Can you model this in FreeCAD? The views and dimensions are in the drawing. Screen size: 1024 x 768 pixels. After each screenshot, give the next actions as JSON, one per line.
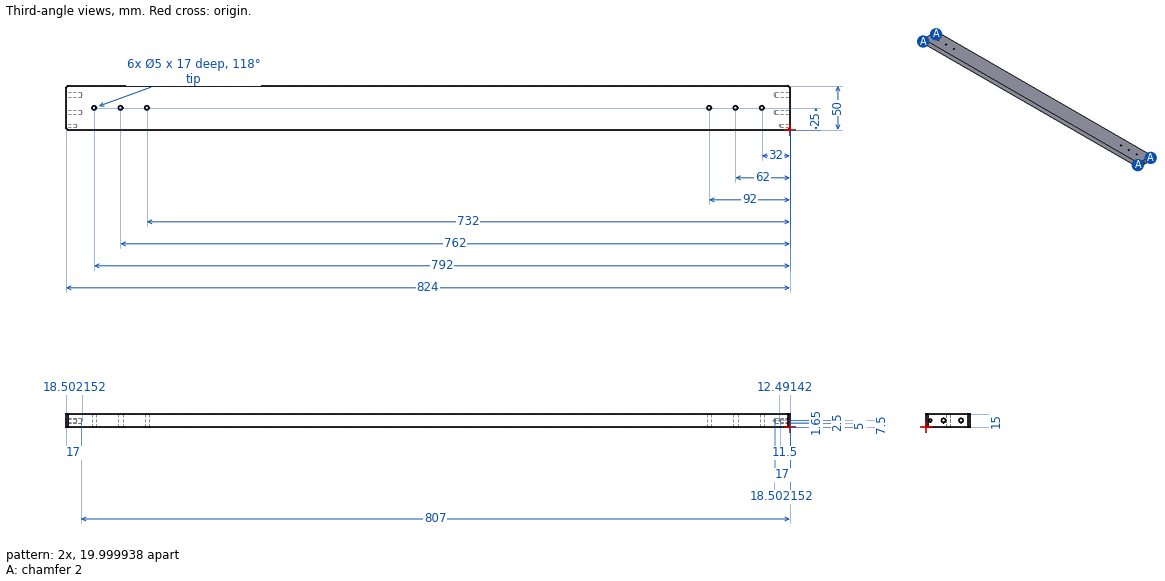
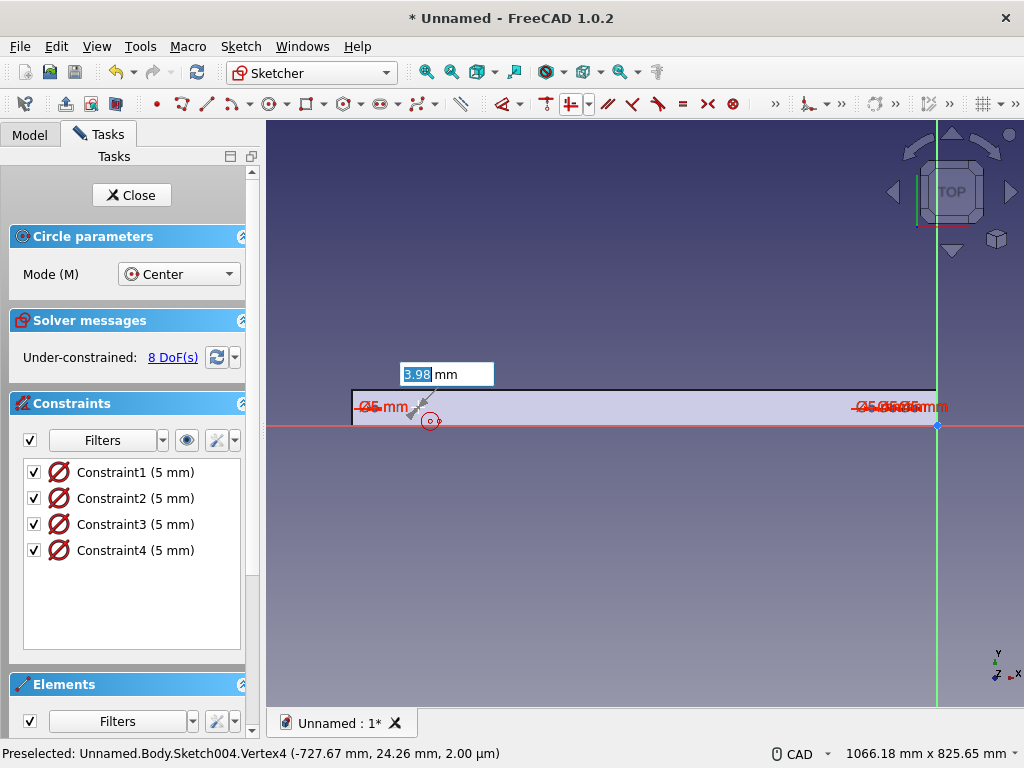
{"action": "type", "text": "5"}
{"action": "key", "text": "Return"}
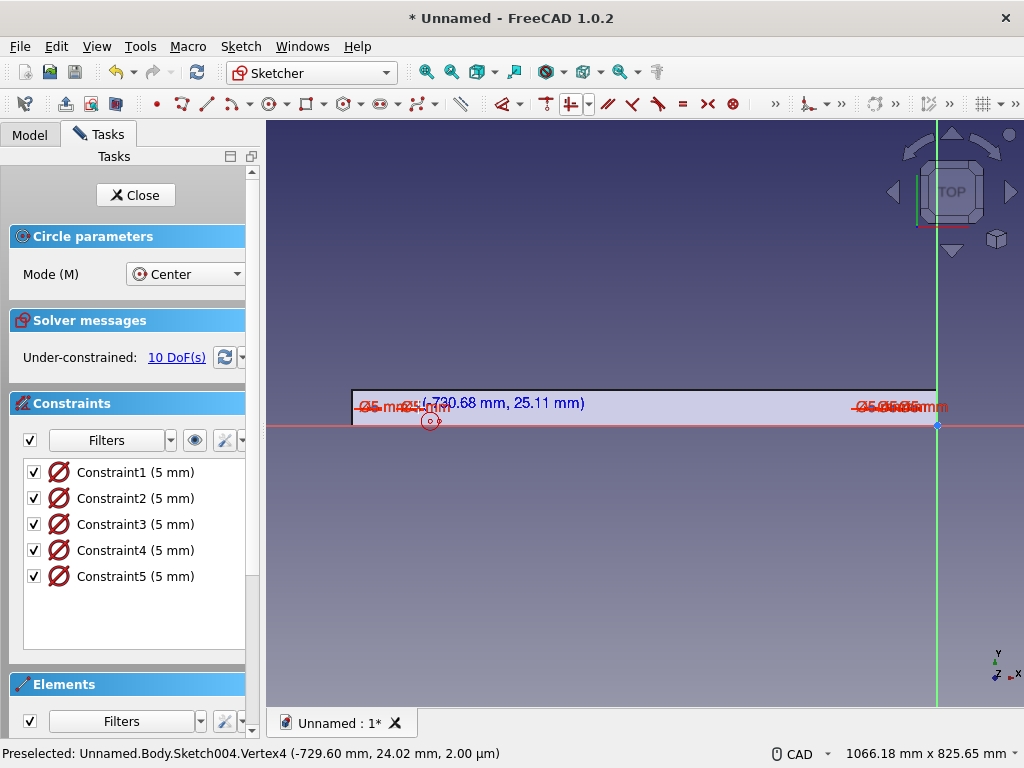
{"action": "scroll", "coordinate": [396, 408], "scroll_direction": "up", "scroll_amount": 13}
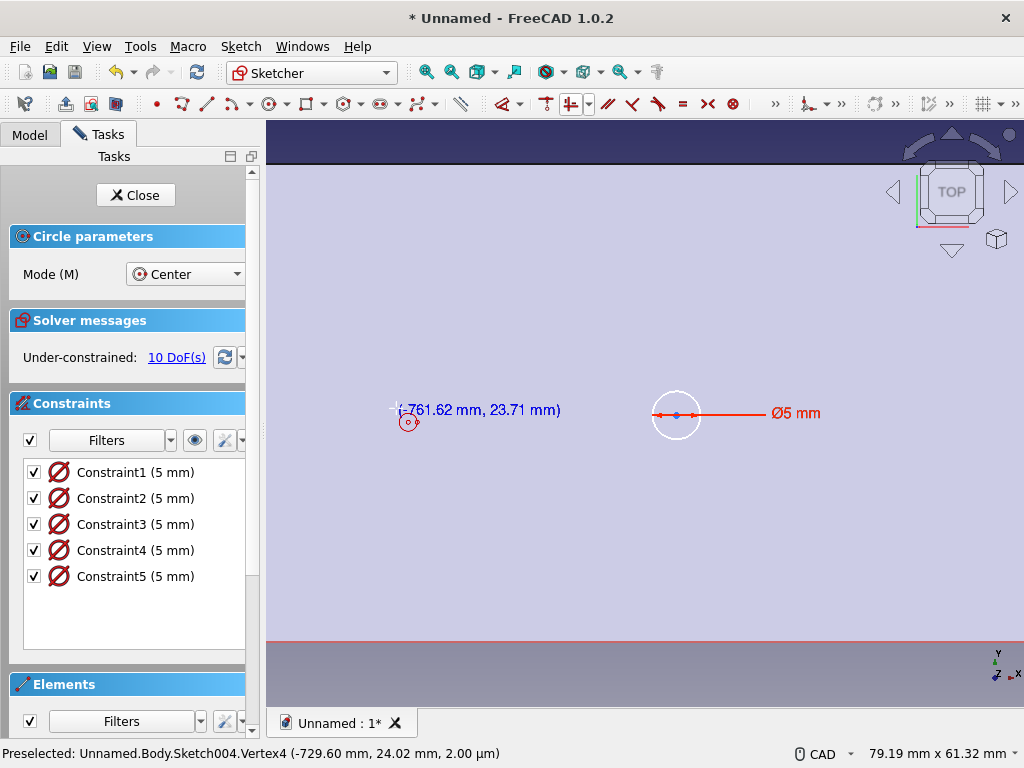
{"action": "scroll", "coordinate": [403, 408], "scroll_direction": "down", "scroll_amount": 15}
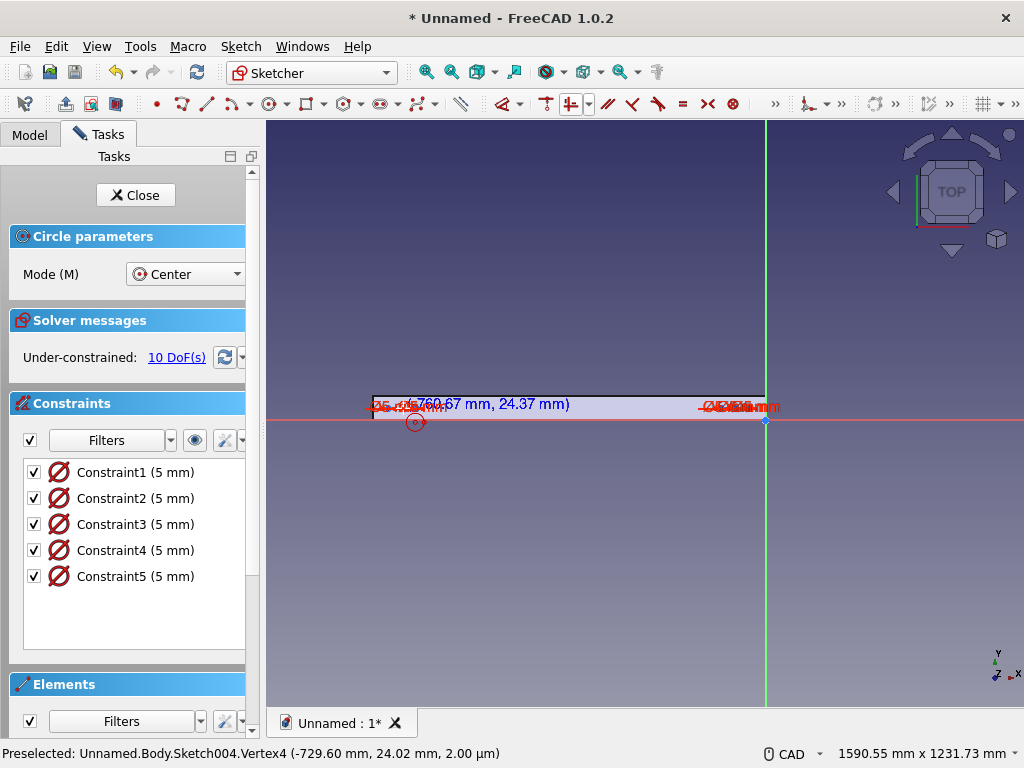
{"action": "scroll", "coordinate": [403, 408], "scroll_direction": "up", "scroll_amount": 2}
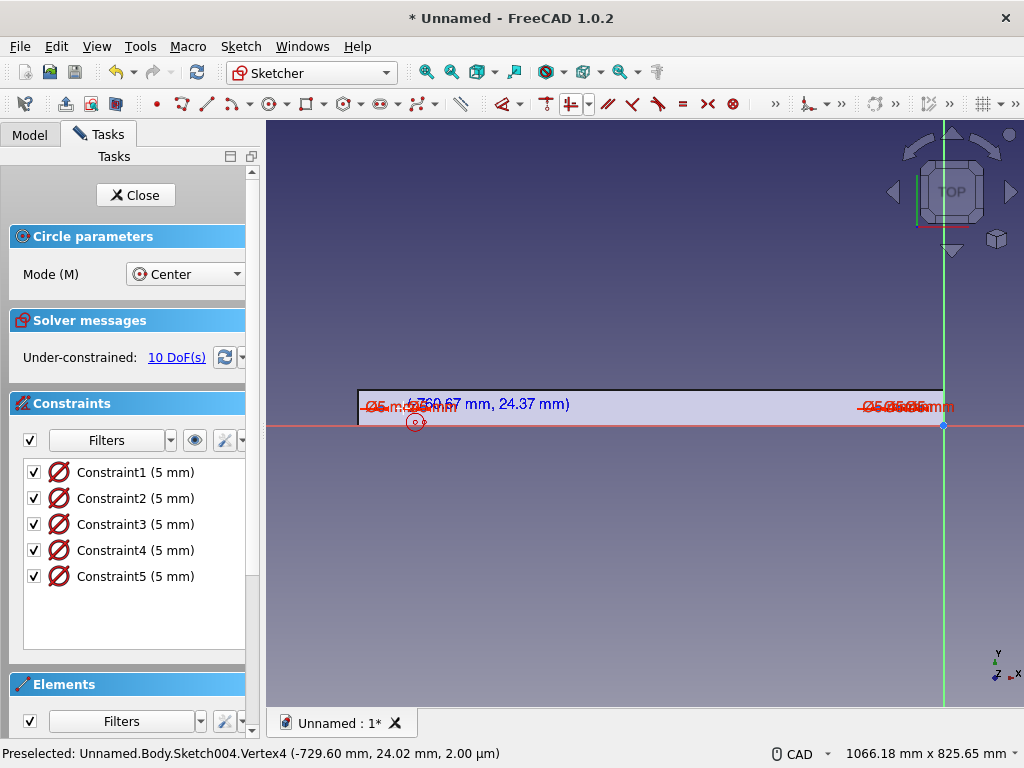
{"action": "left_click", "coordinate": [402, 408]}
{"action": "mouse_move", "coordinate": [403, 407]}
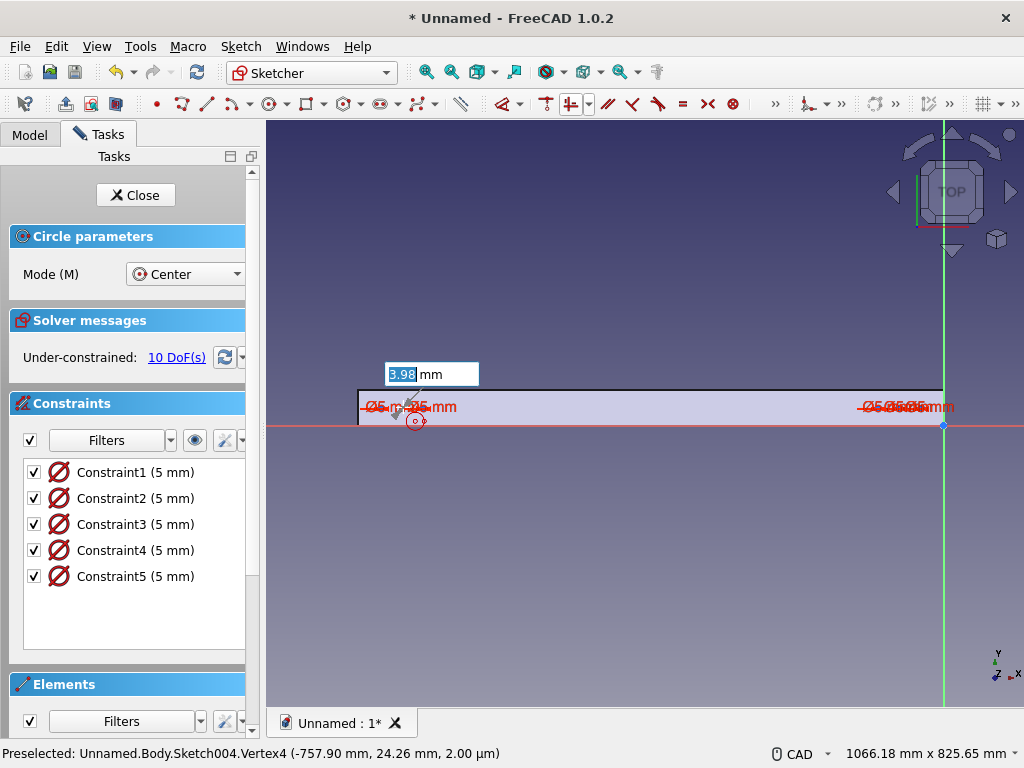
{"action": "type", "text": "5"}
{"action": "key", "text": "Return"}
{"action": "key", "text": "Escape"}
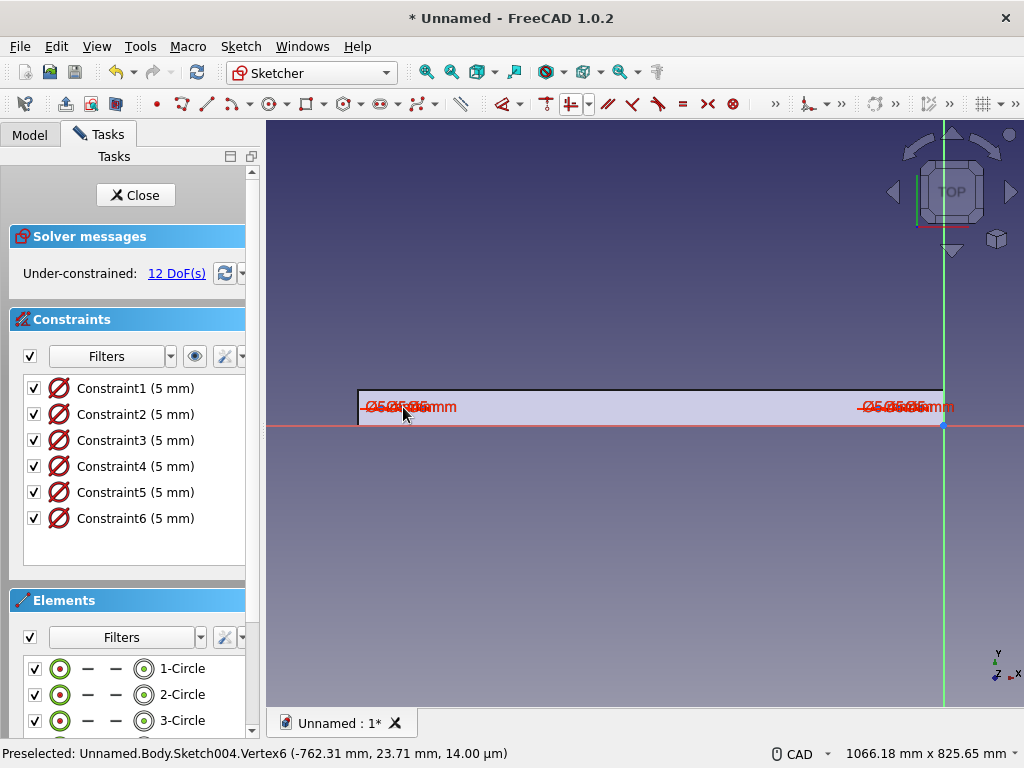
{"action": "left_click", "coordinate": [381, 409]}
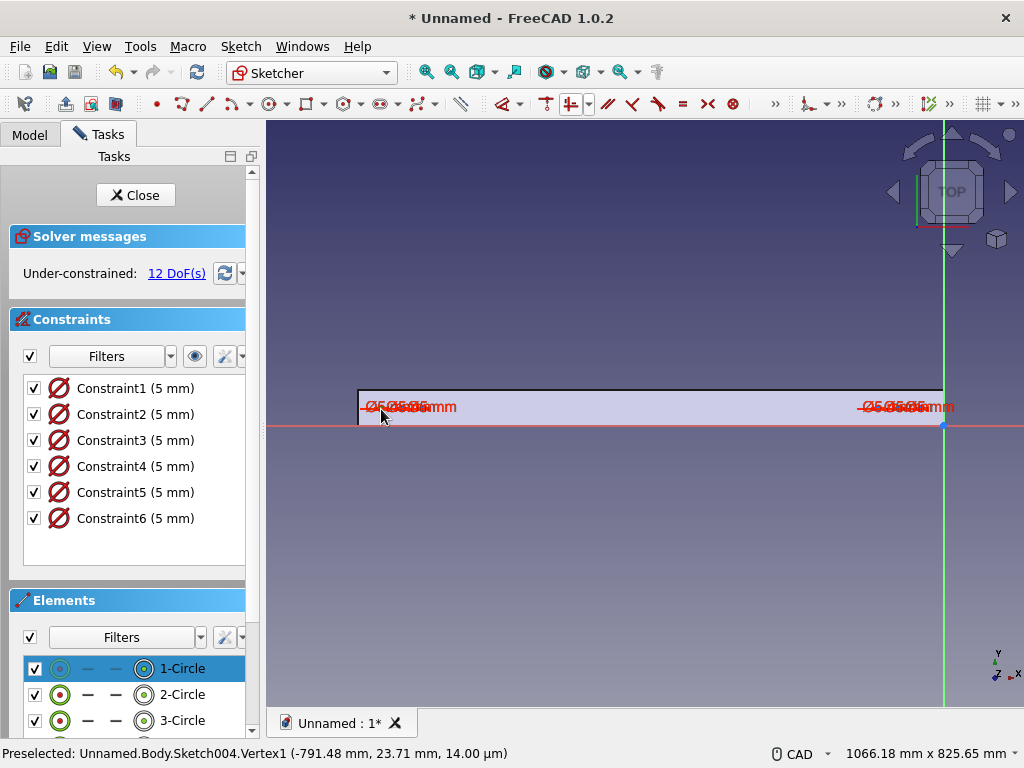
{"action": "scroll", "coordinate": [404, 408], "scroll_direction": "down", "scroll_amount": 2}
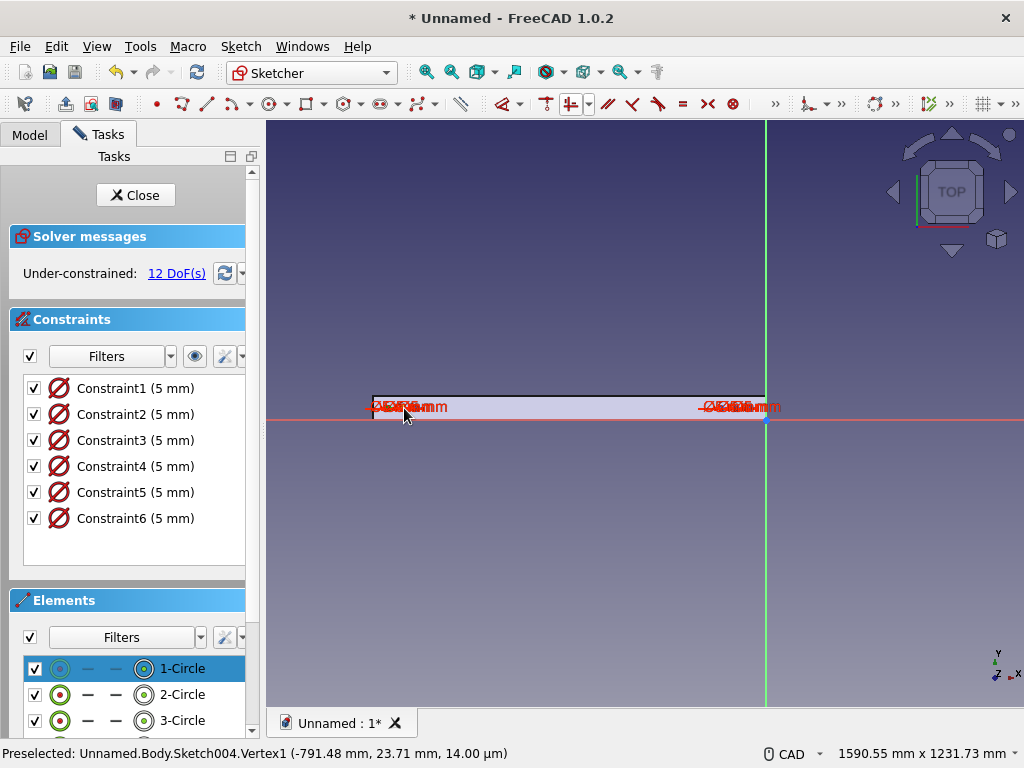
{"action": "left_click", "coordinate": [751, 409]}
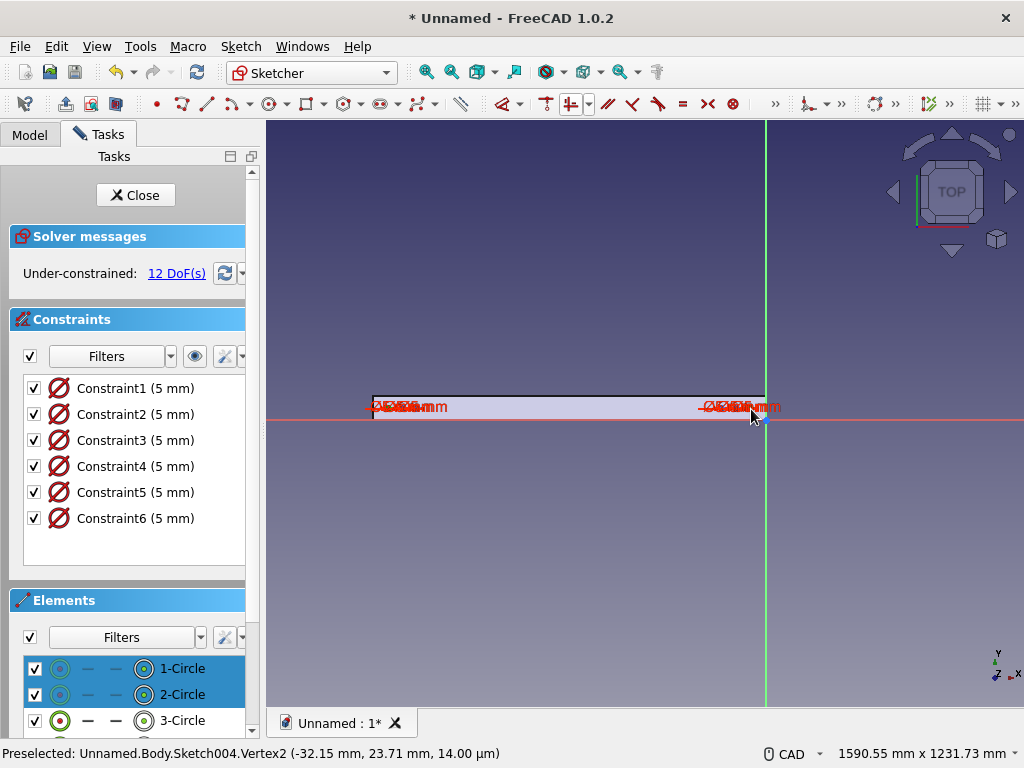
{"action": "left_click", "coordinate": [588, 104]}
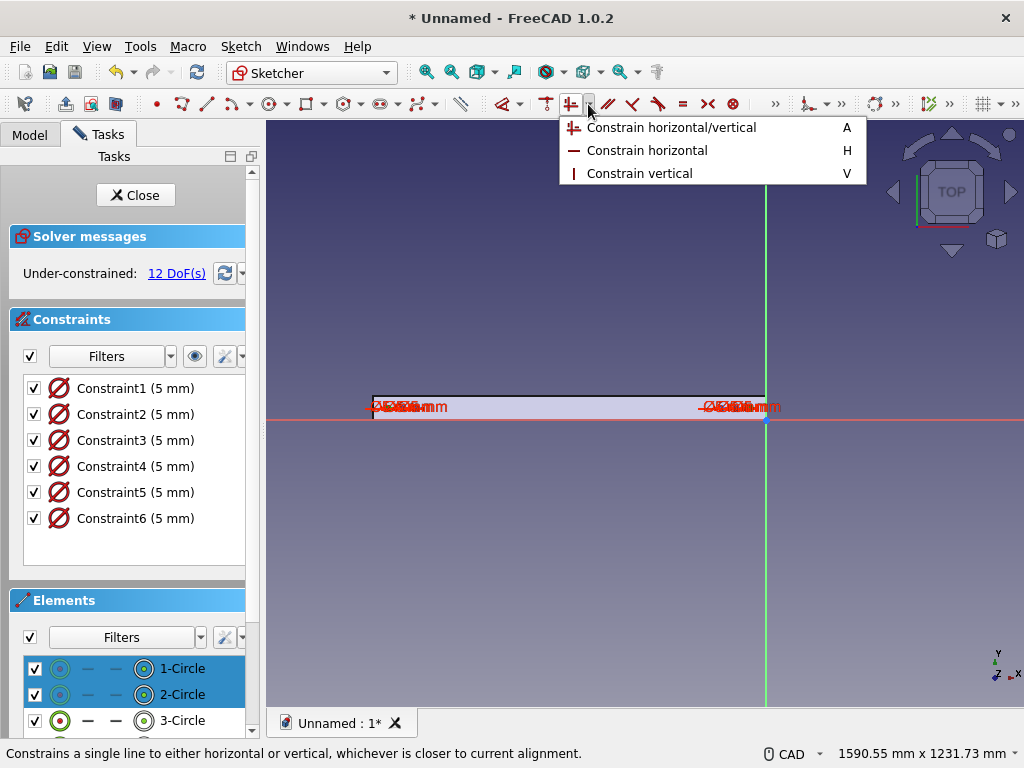
{"action": "left_click", "coordinate": [713, 150]}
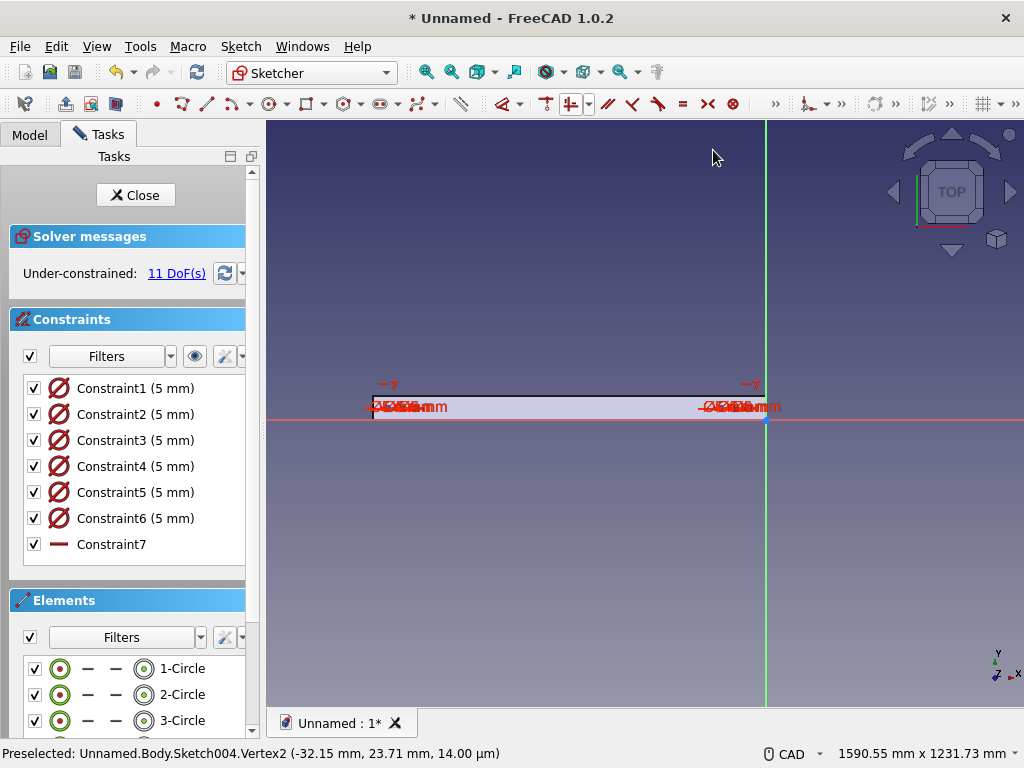
{"action": "left_click", "coordinate": [751, 409]}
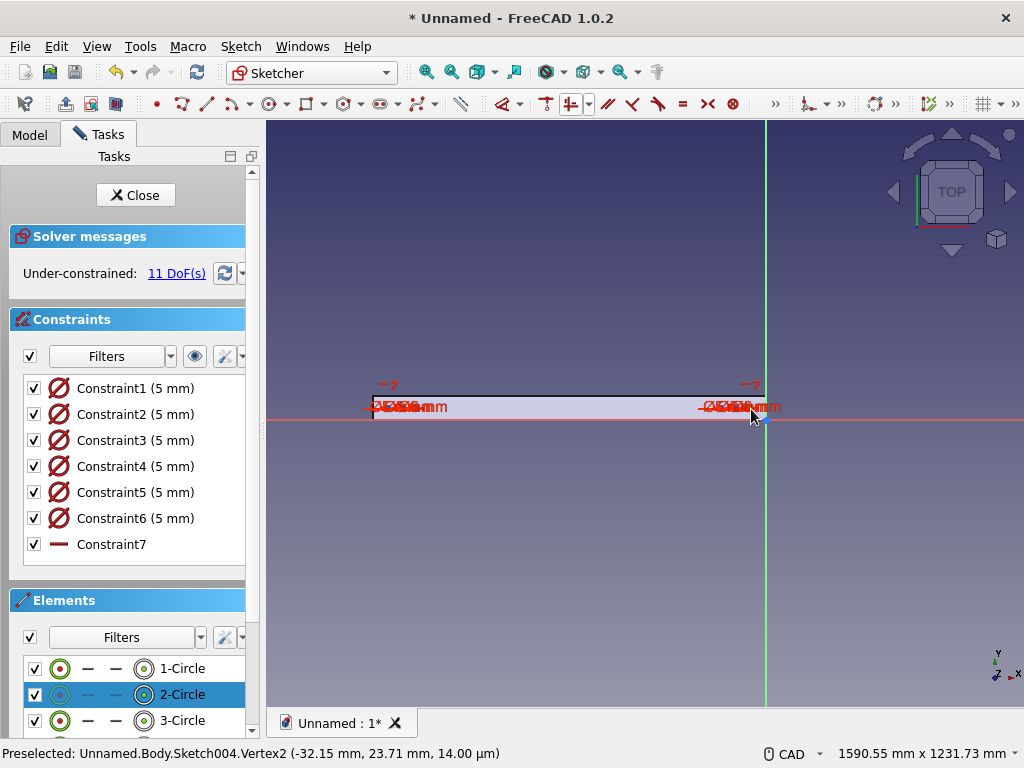
{"action": "left_click", "coordinate": [736, 409]}